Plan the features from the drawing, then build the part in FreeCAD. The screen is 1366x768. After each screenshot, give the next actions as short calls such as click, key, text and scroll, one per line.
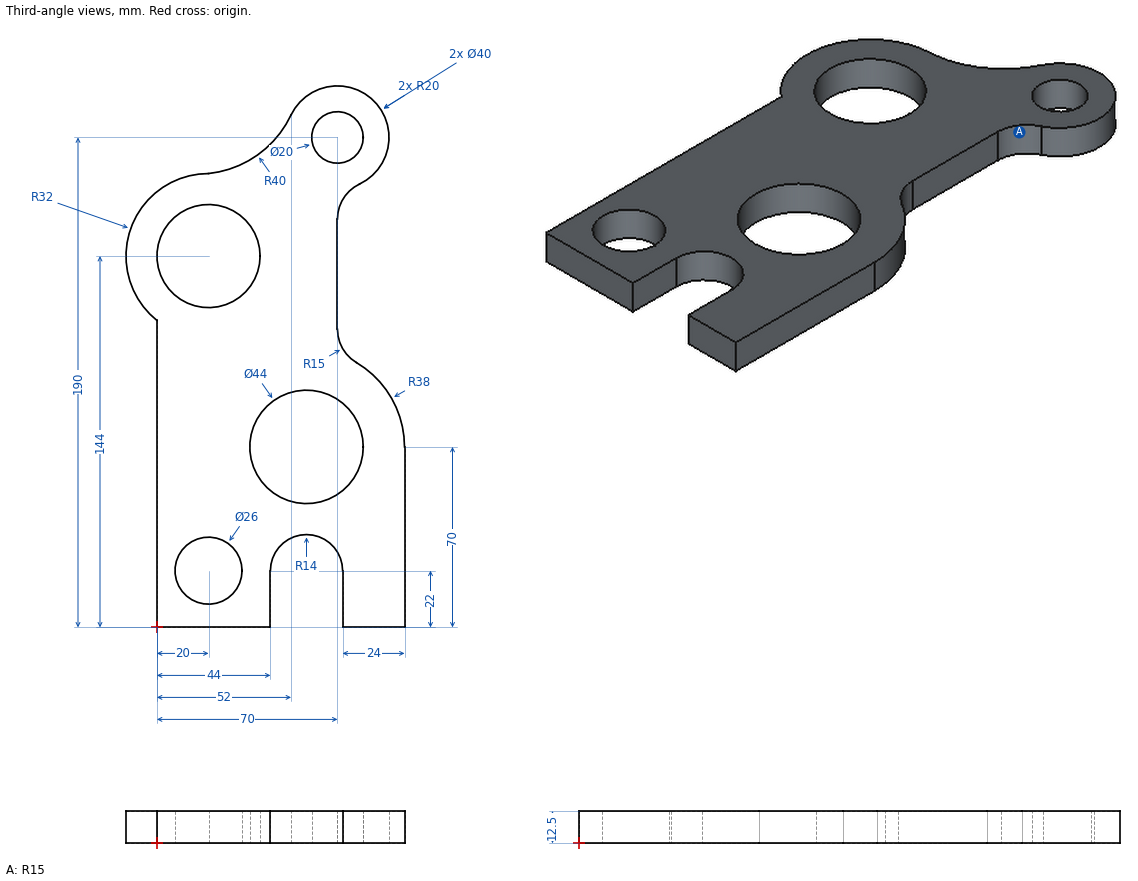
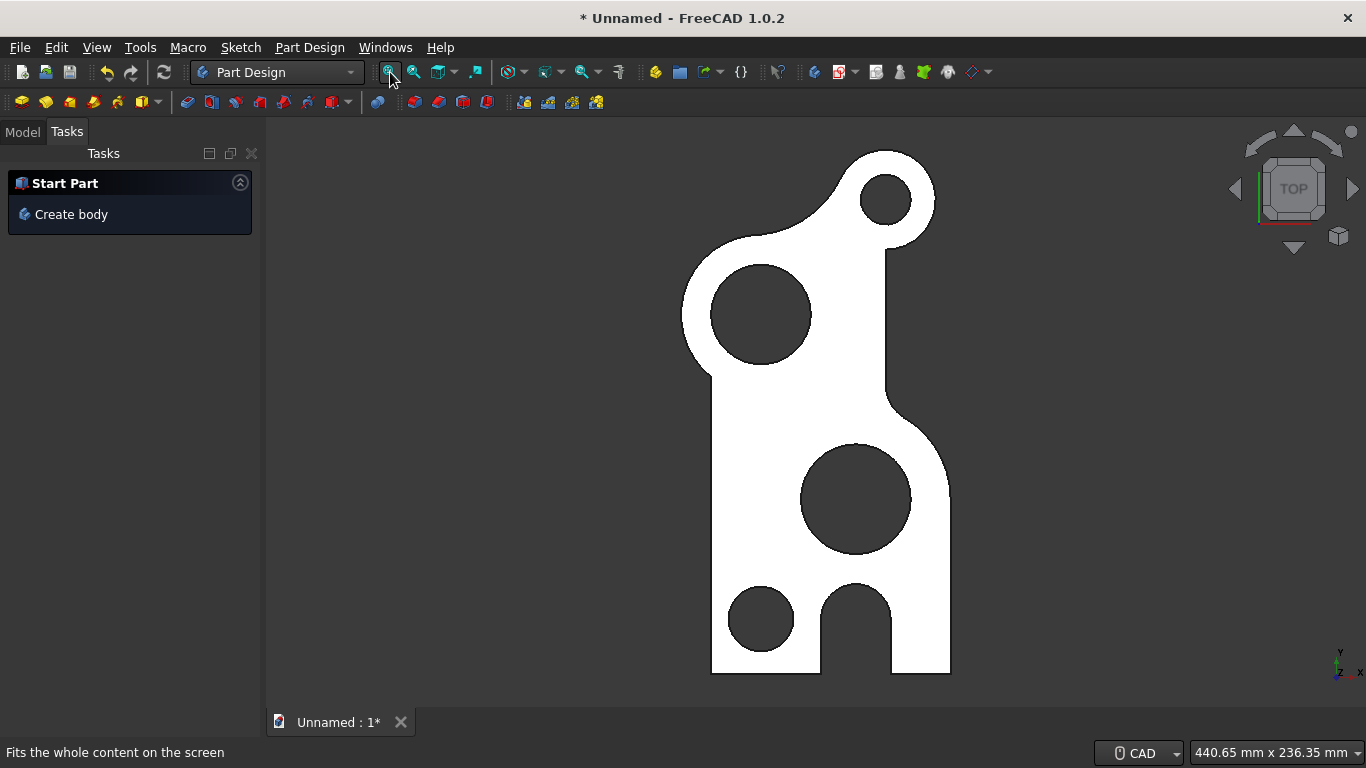
key(1)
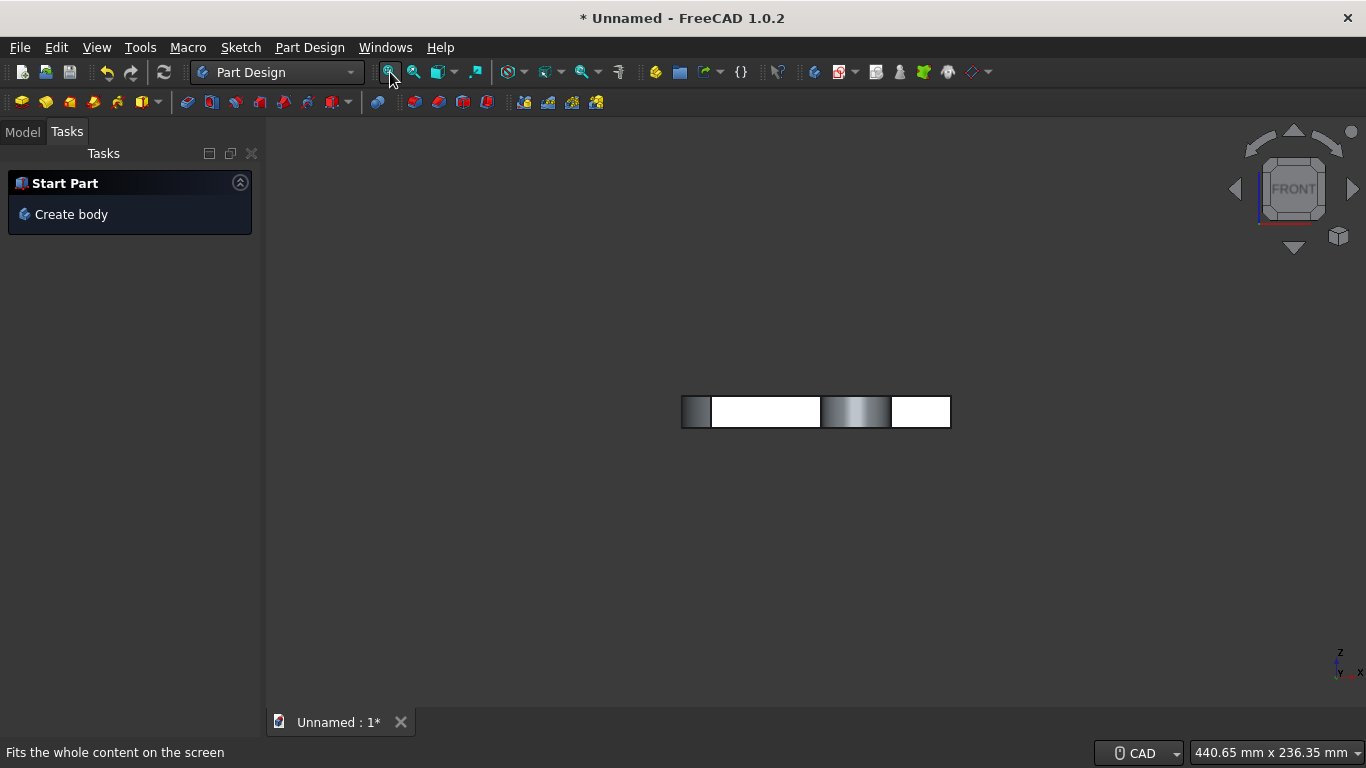
click(390, 72)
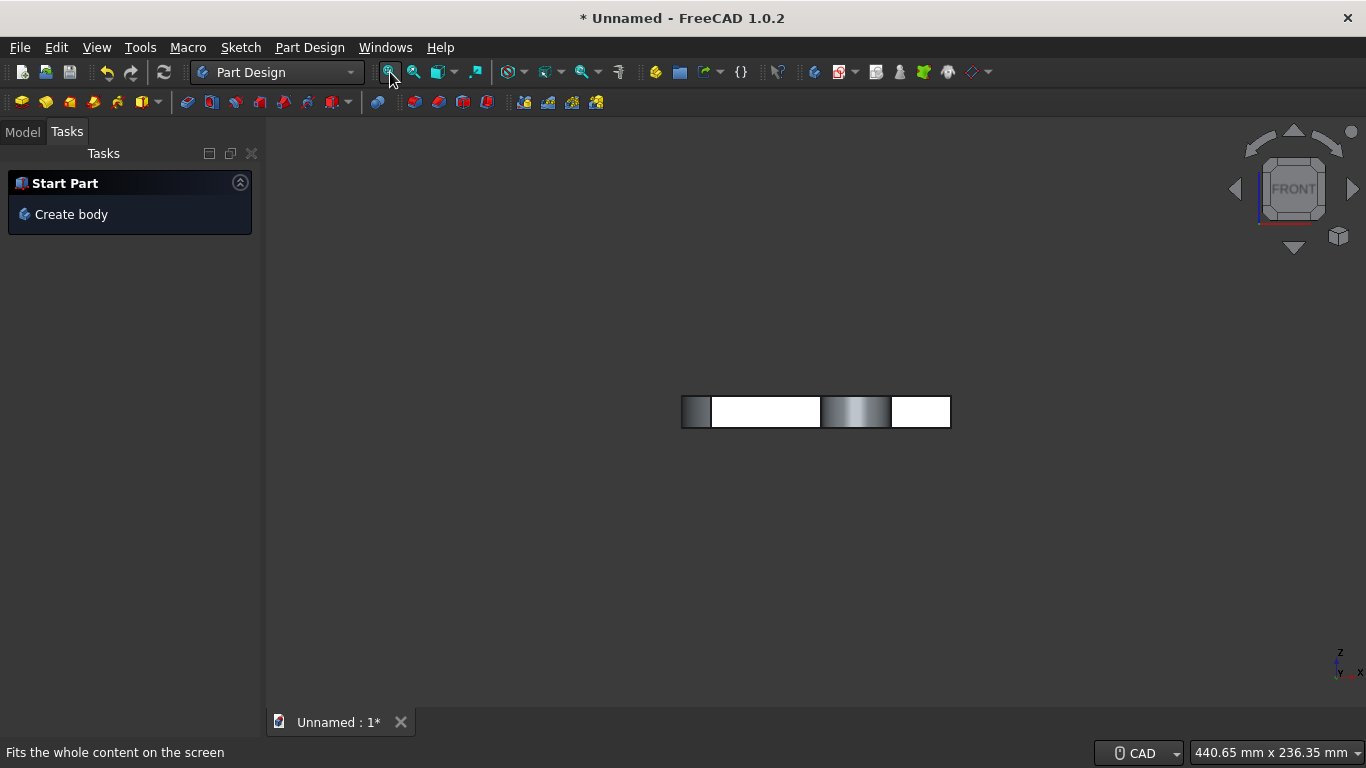
key(3)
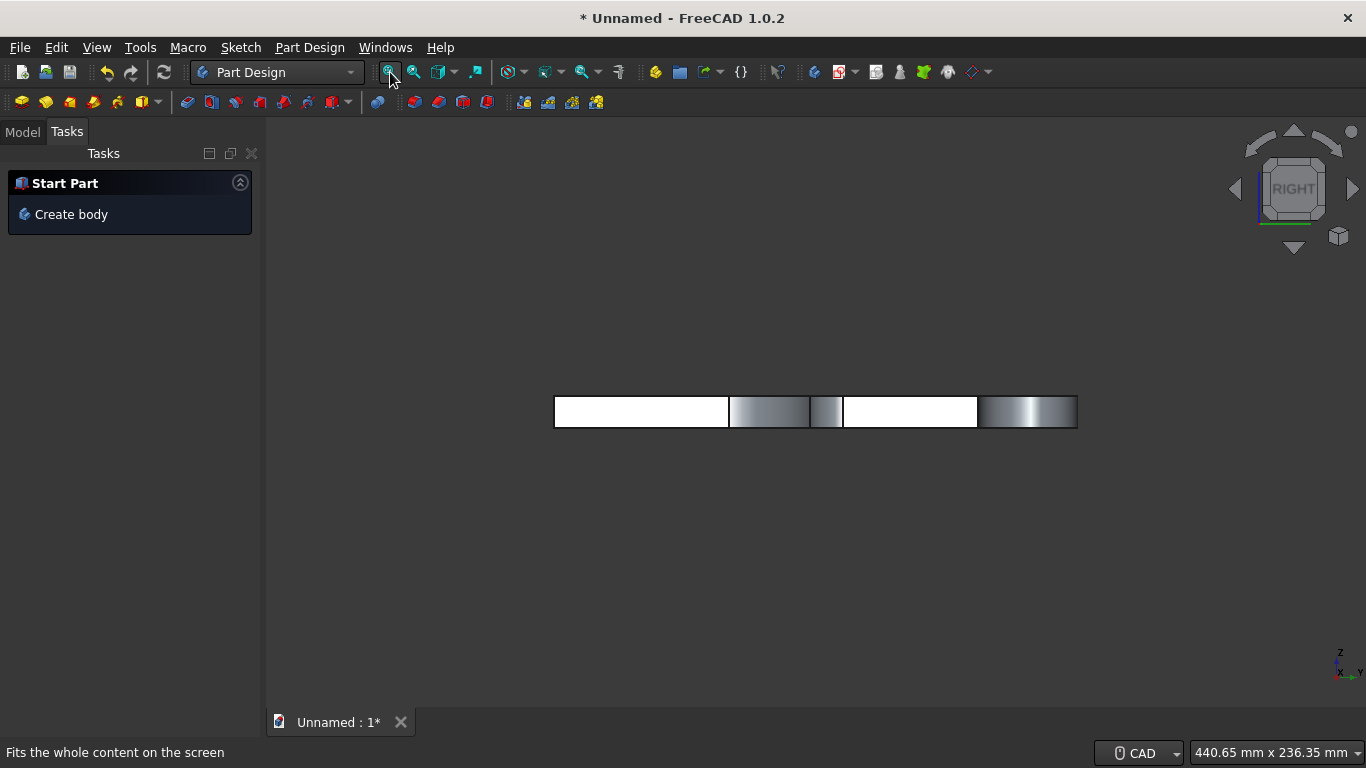
key(5)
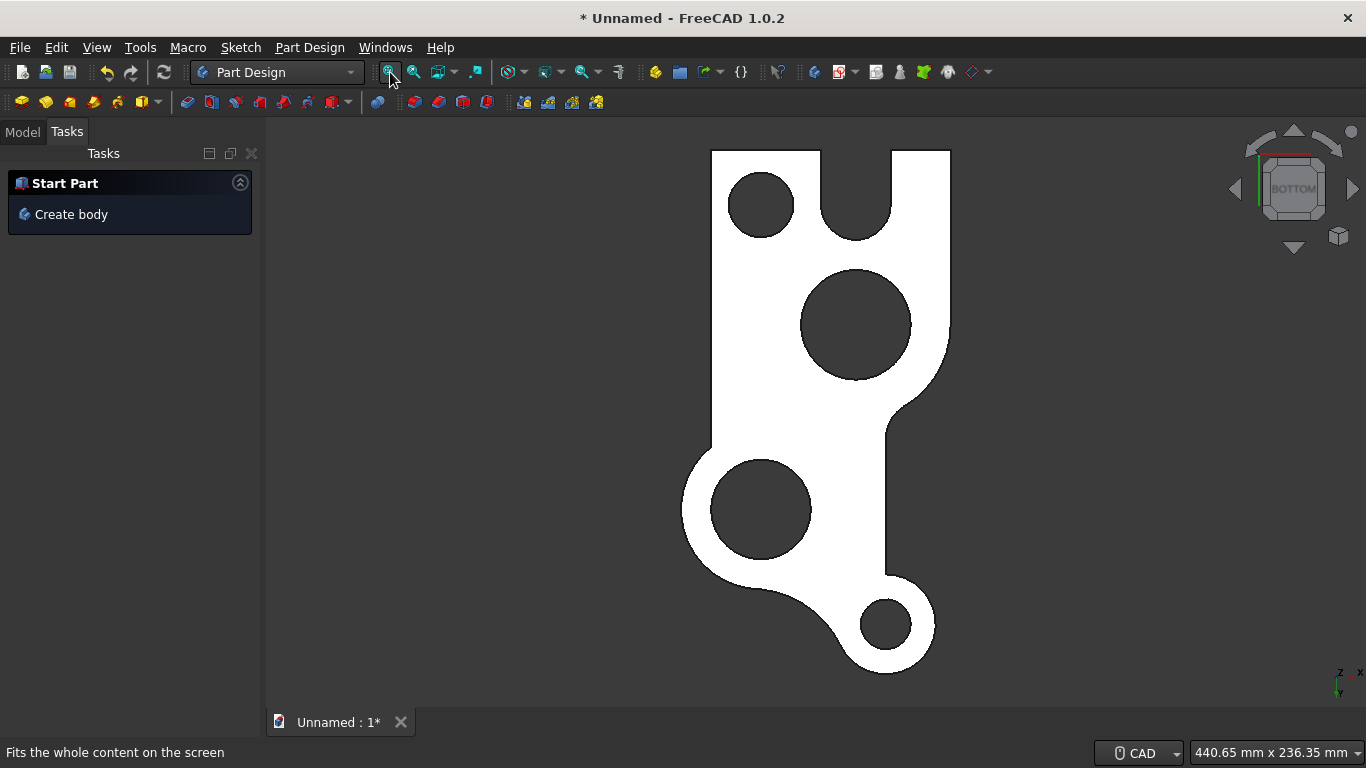
key(4)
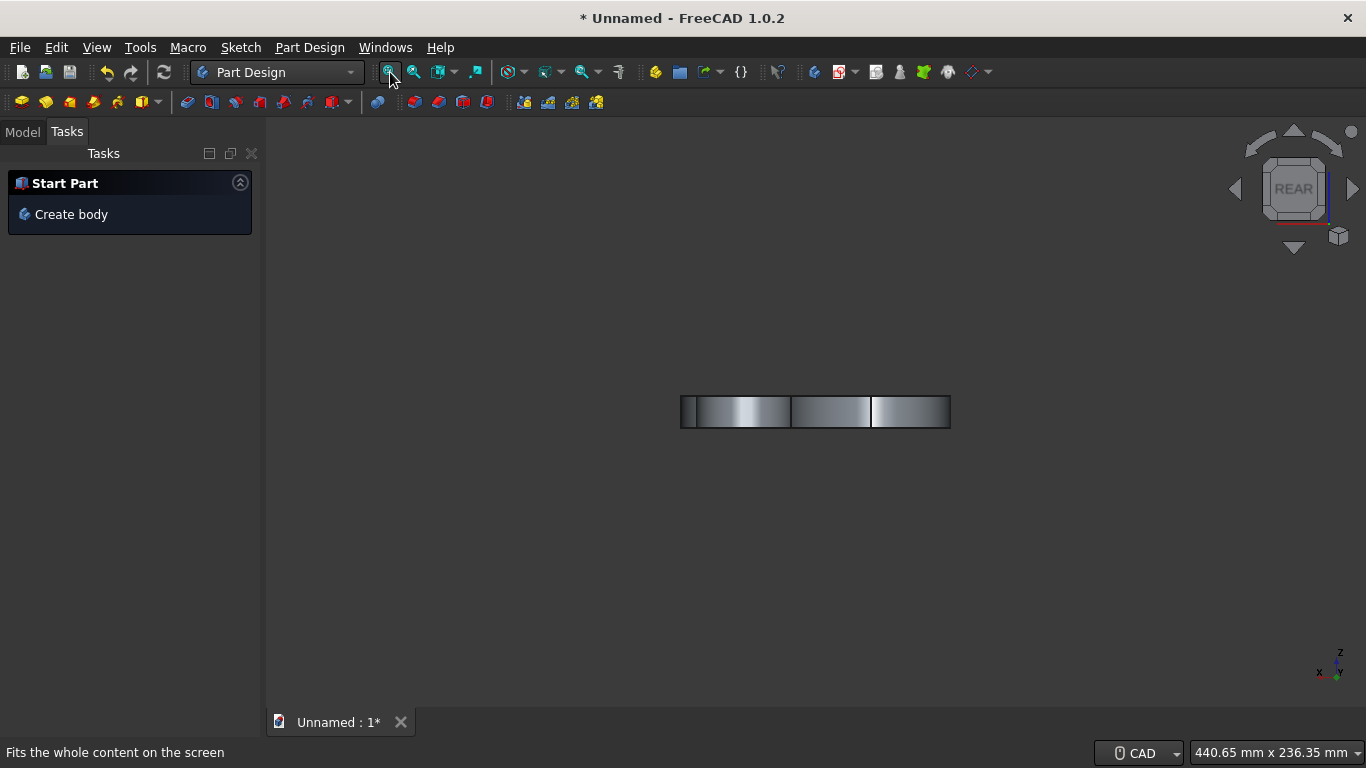
click(390, 72)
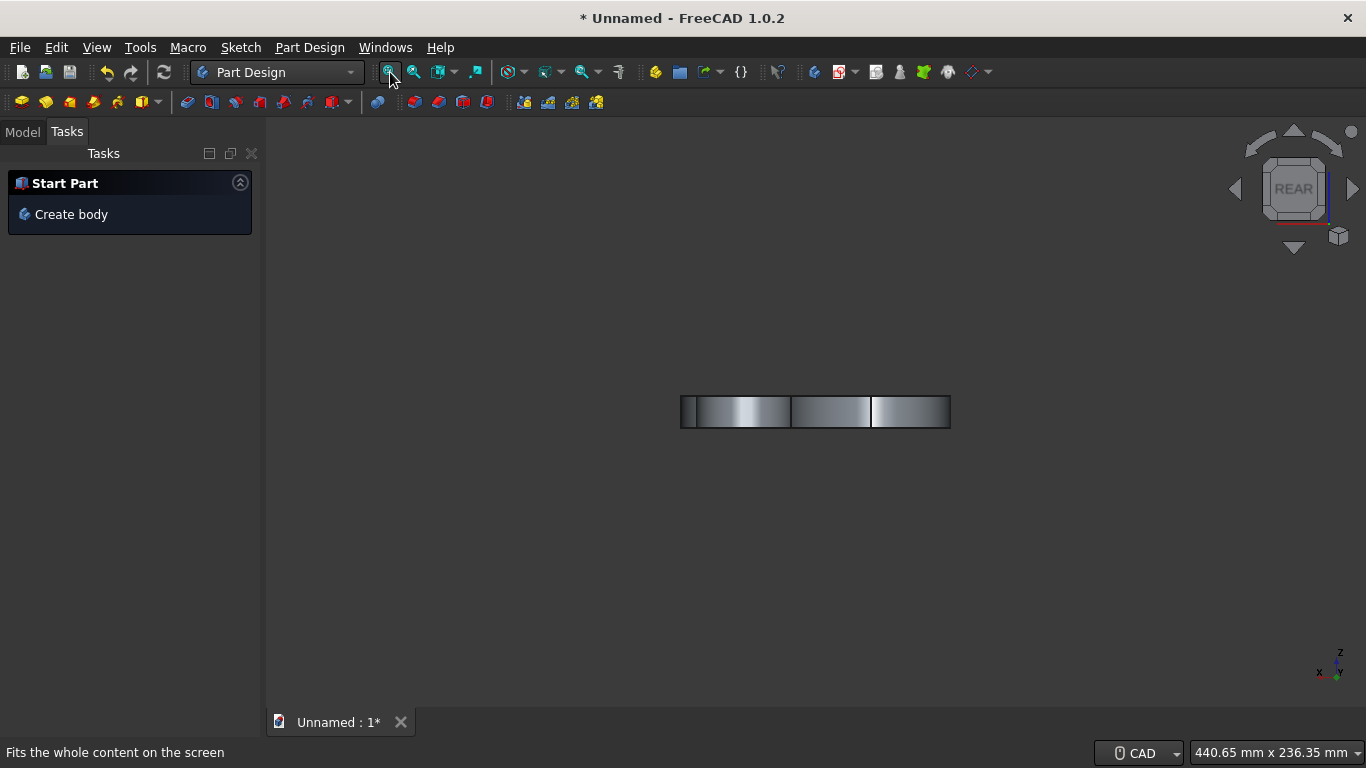
key(6)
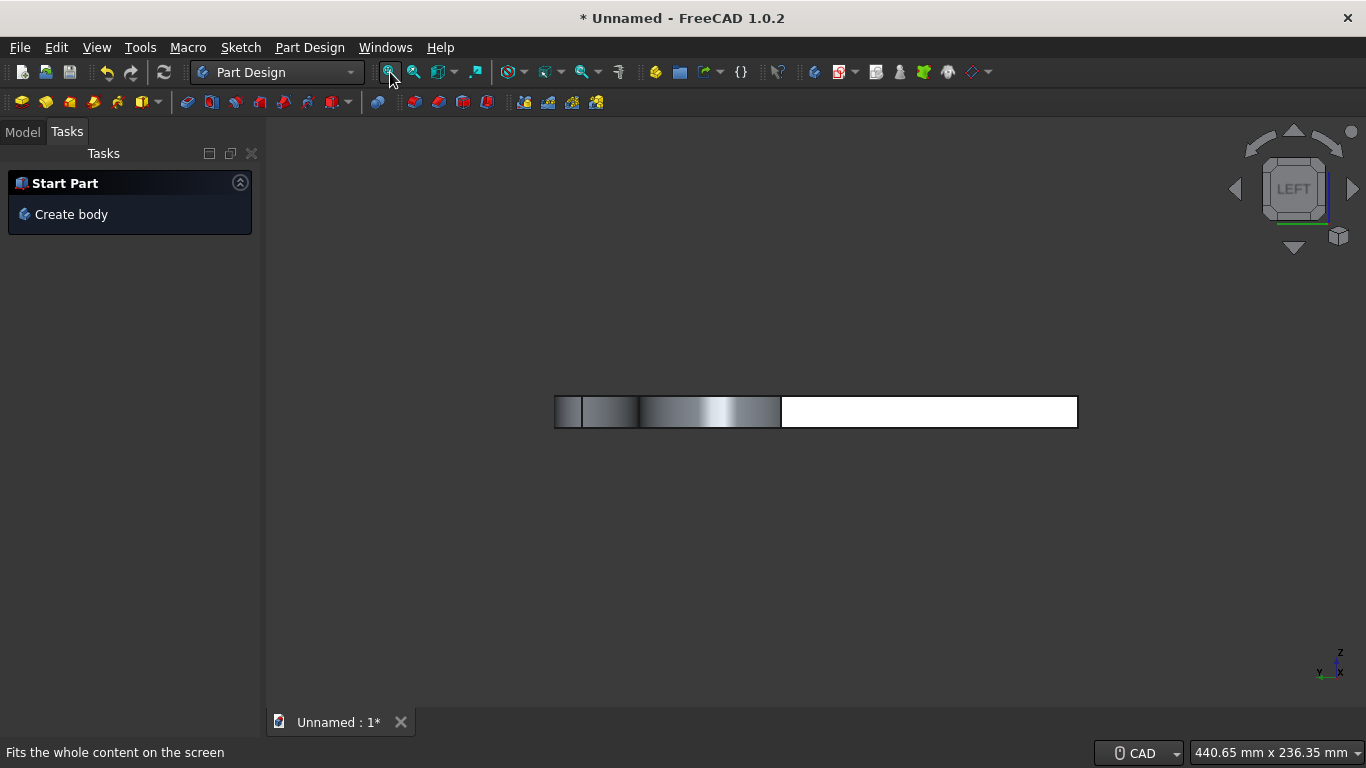
key(v)
key(3)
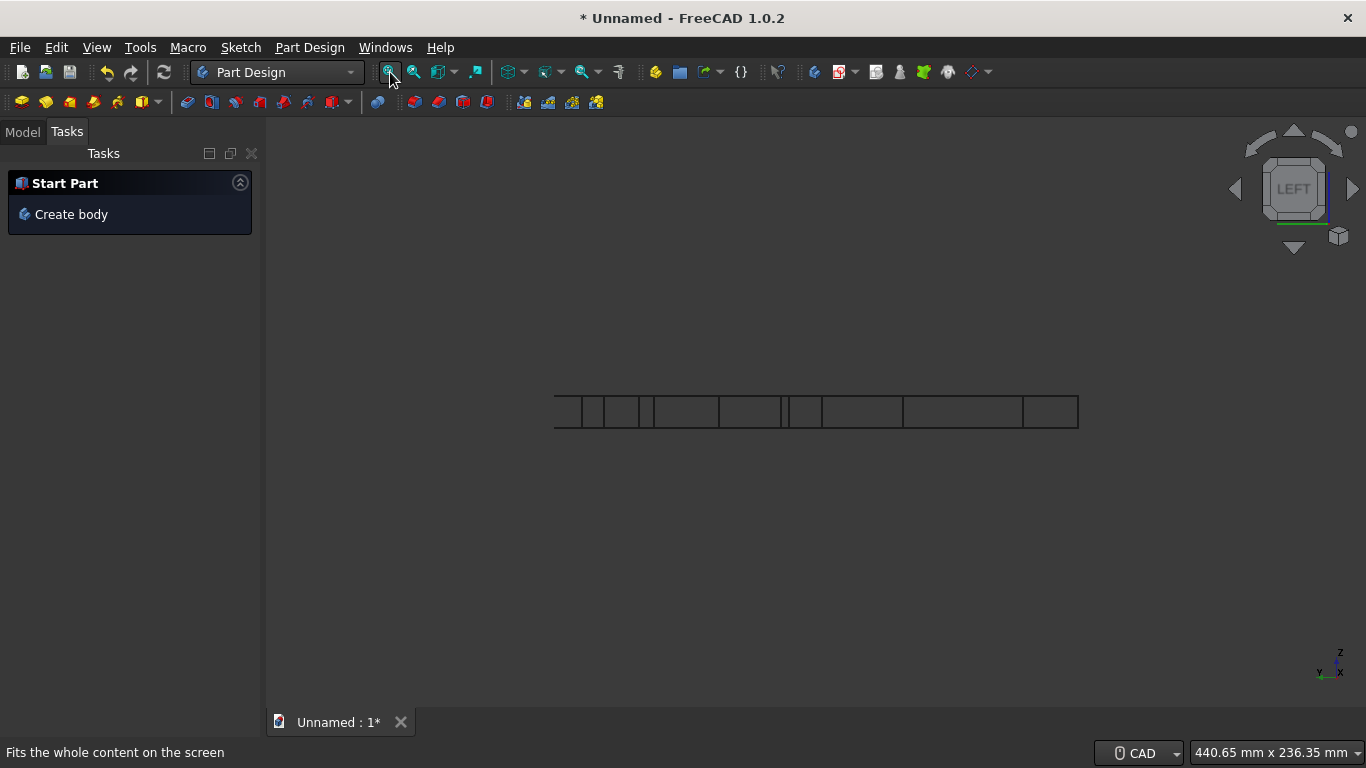
key(0)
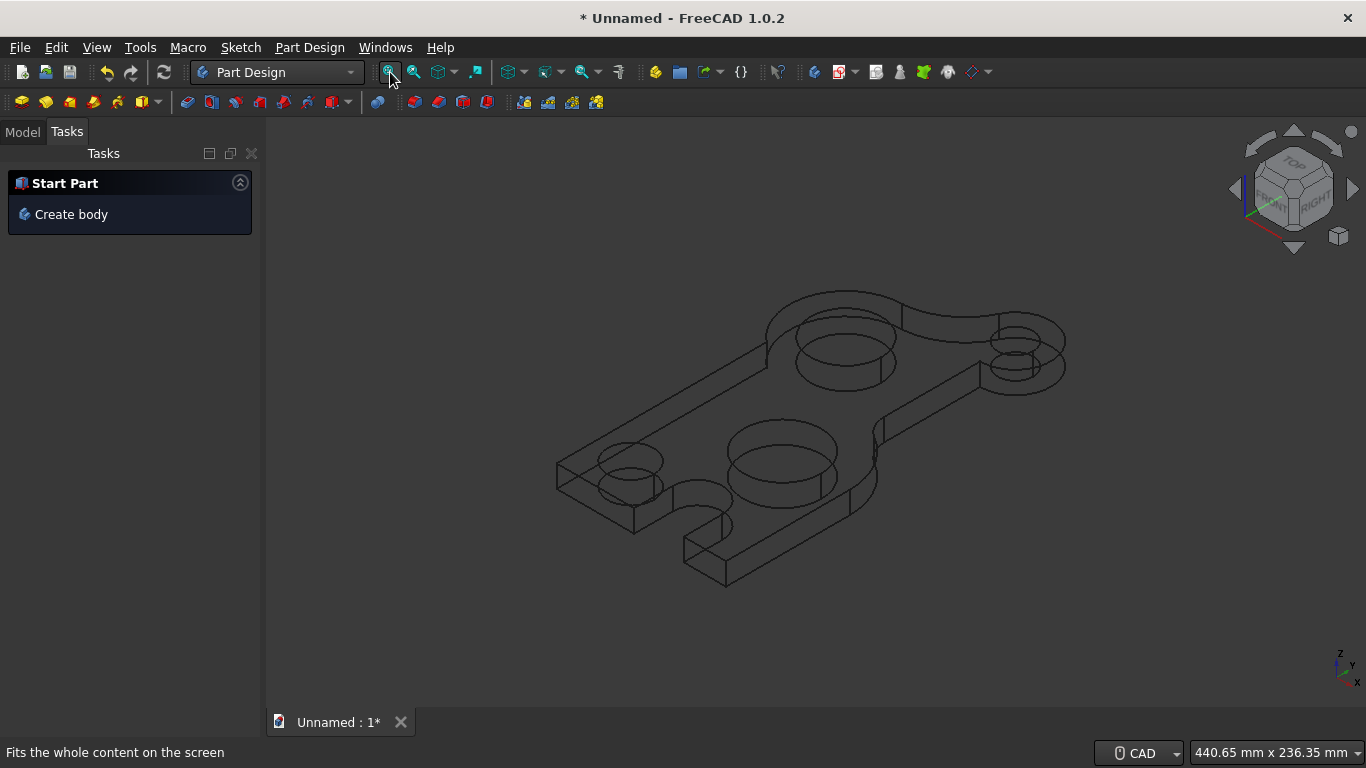
click(980, 373)